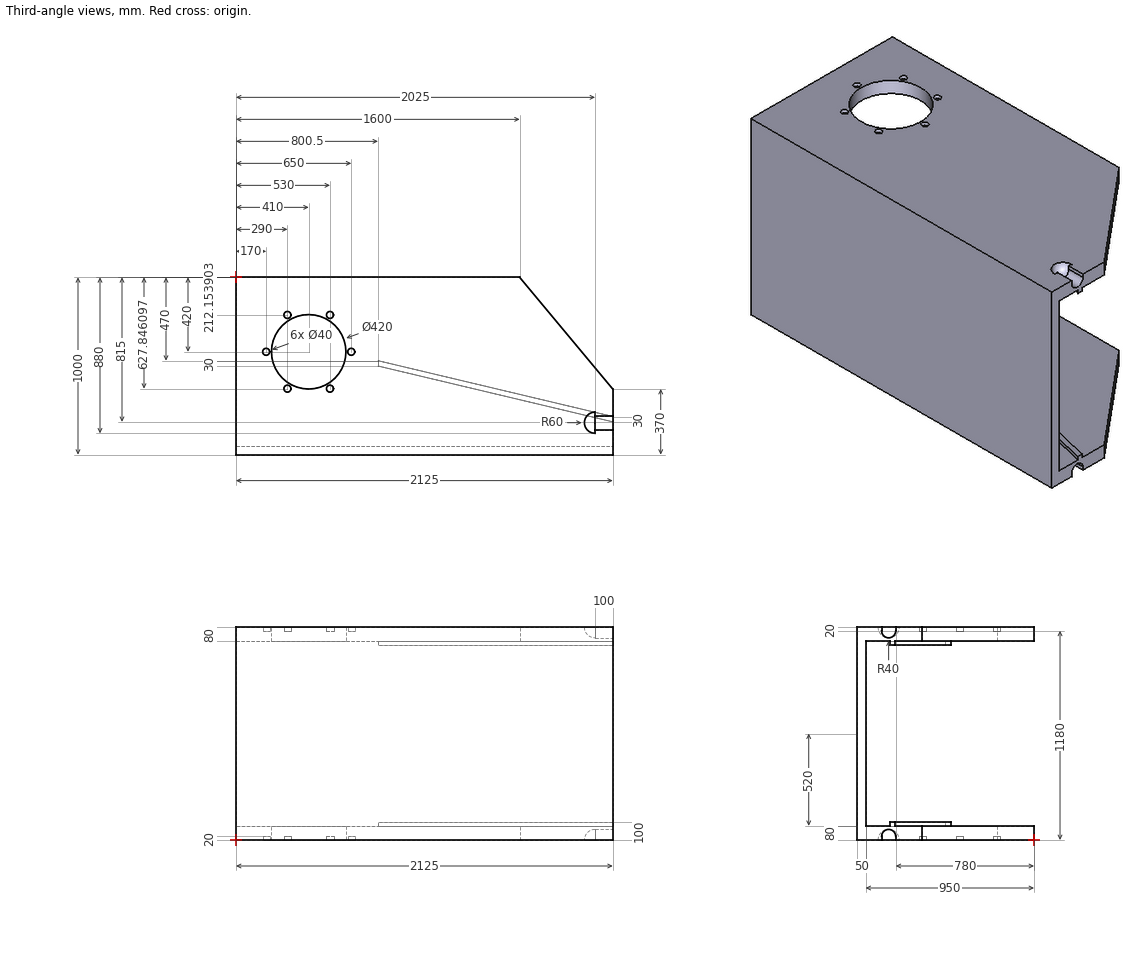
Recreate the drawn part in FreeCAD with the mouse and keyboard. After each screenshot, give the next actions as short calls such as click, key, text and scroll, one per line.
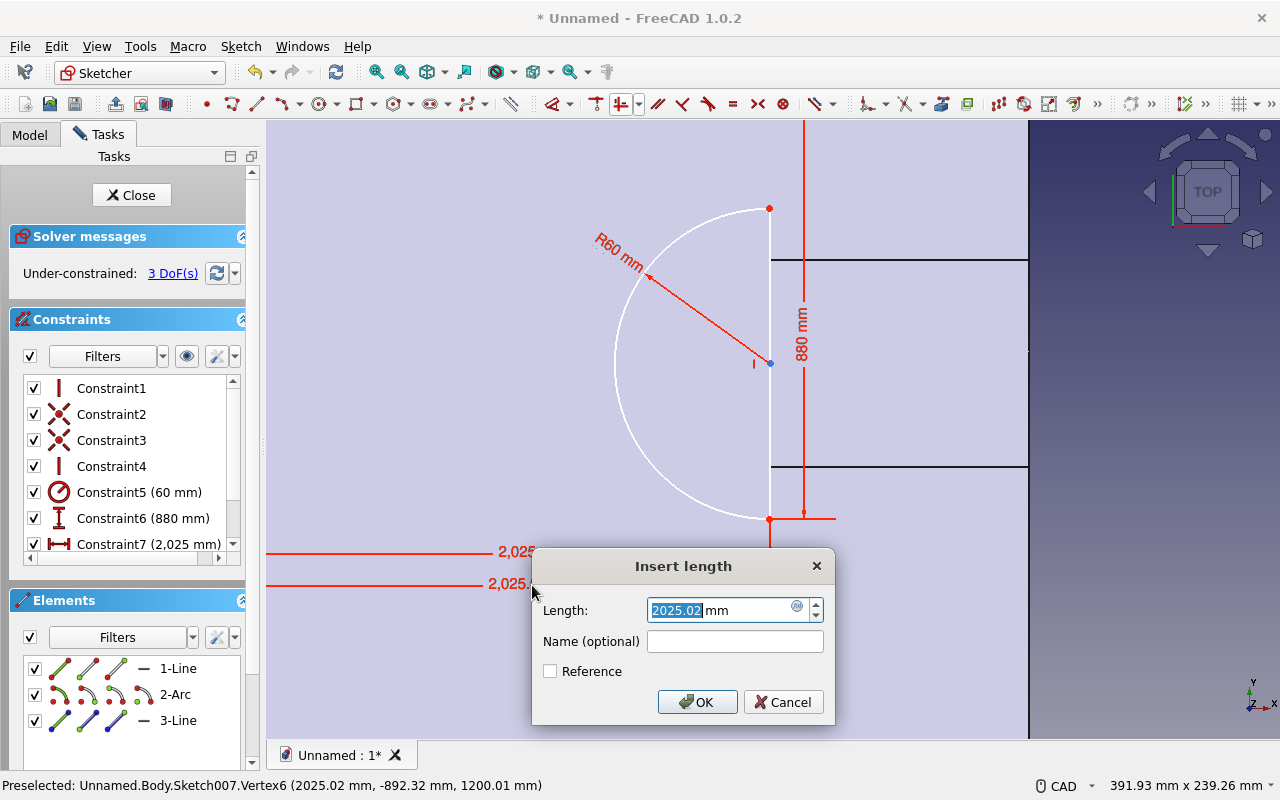
text(2025)
key(Return)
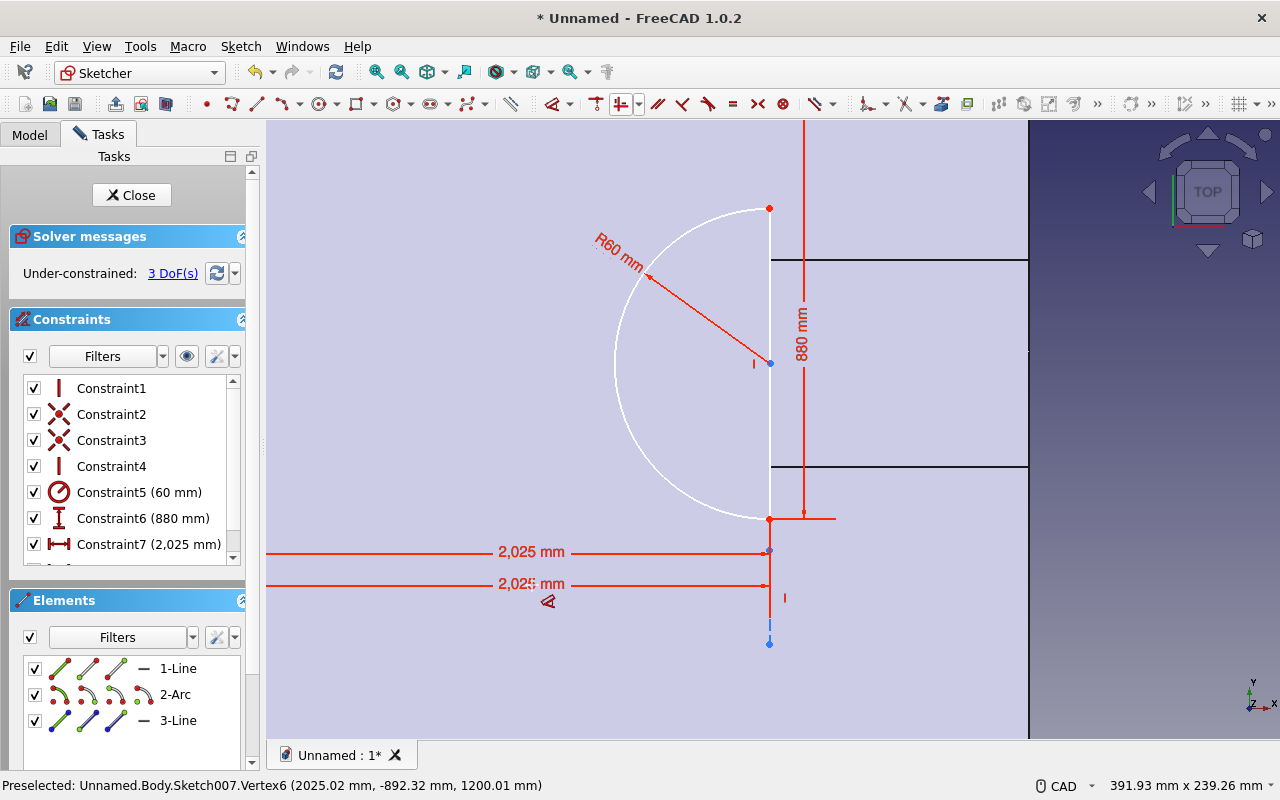
click(770, 364)
click(532, 398)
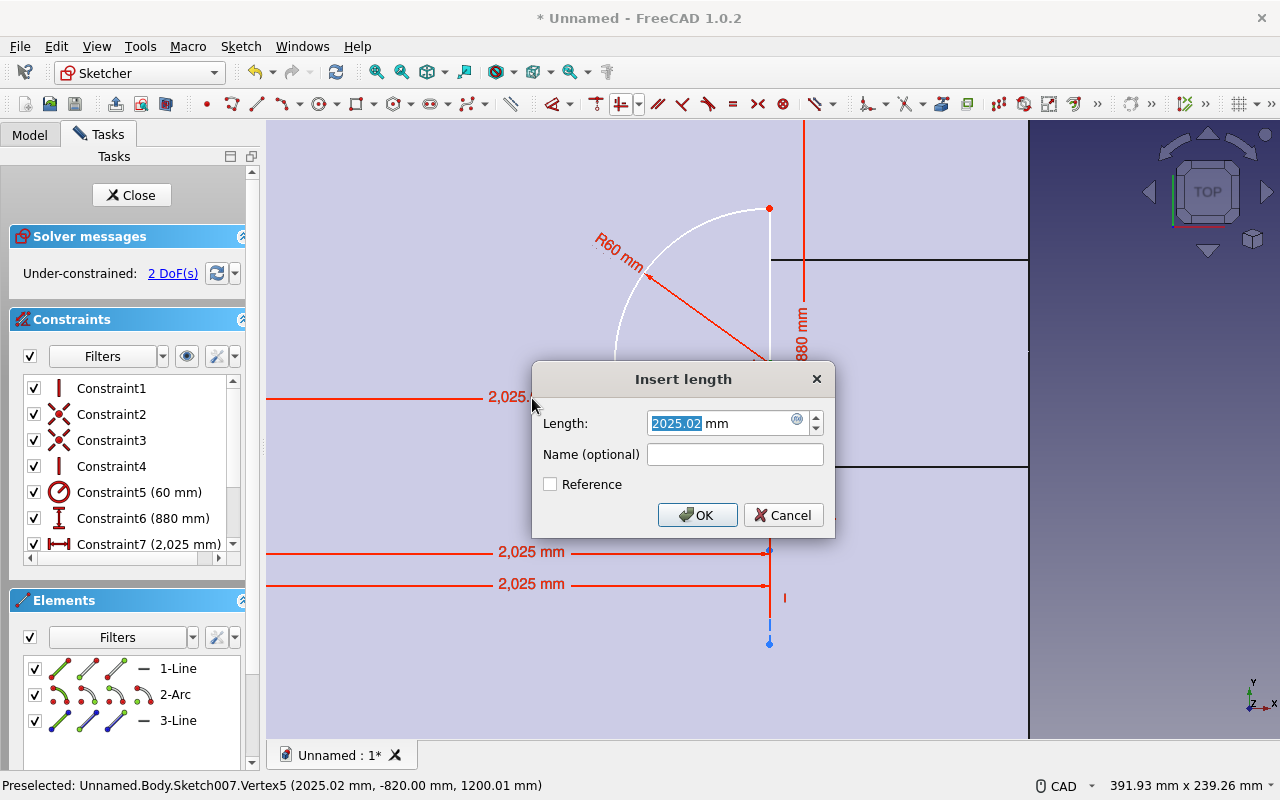
text(2025)
key(Return)
key(Escape)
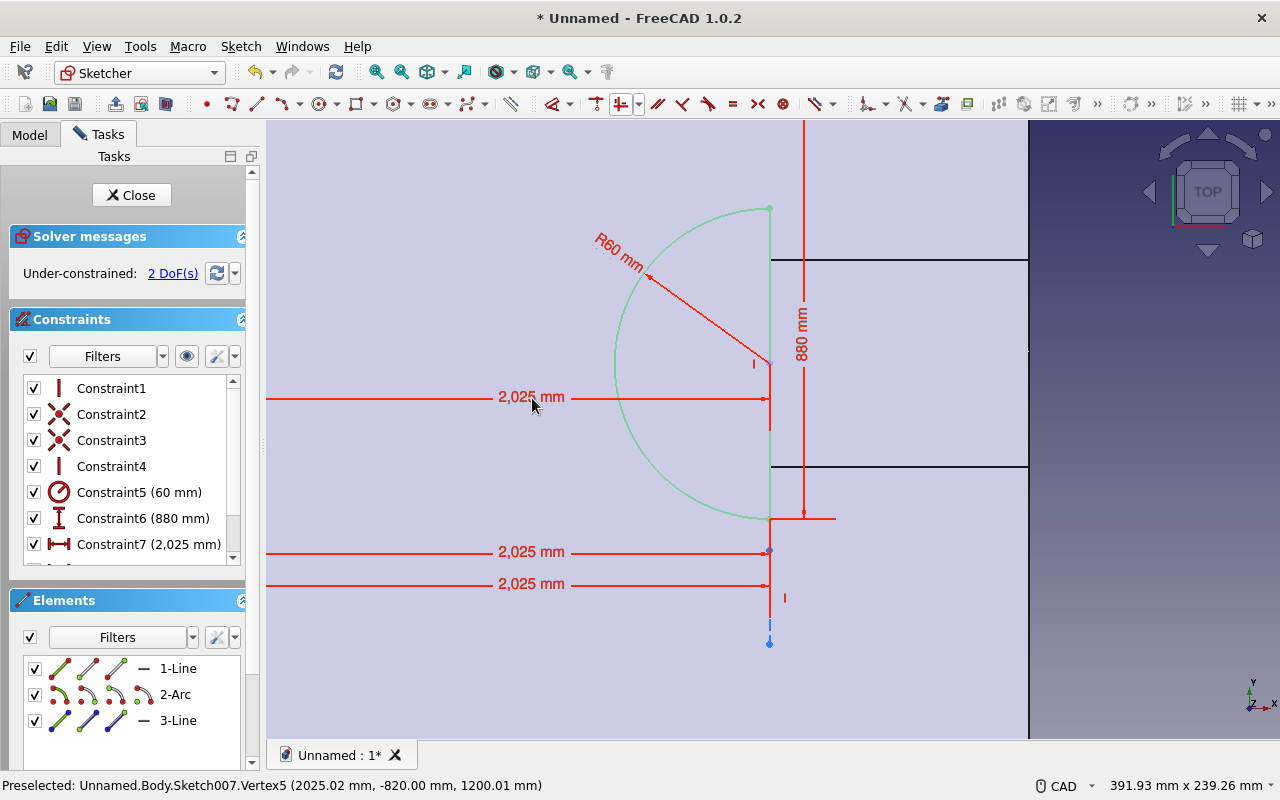
click(132, 195)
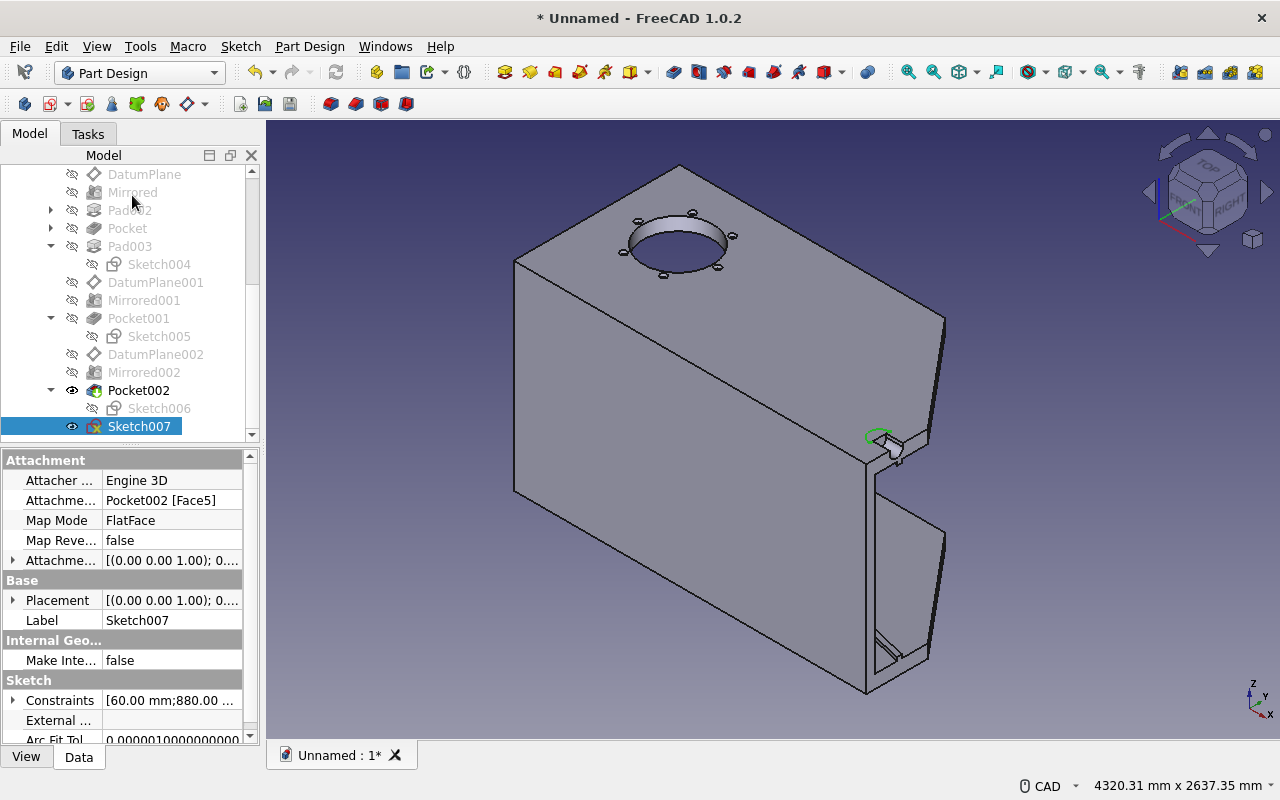
click(724, 72)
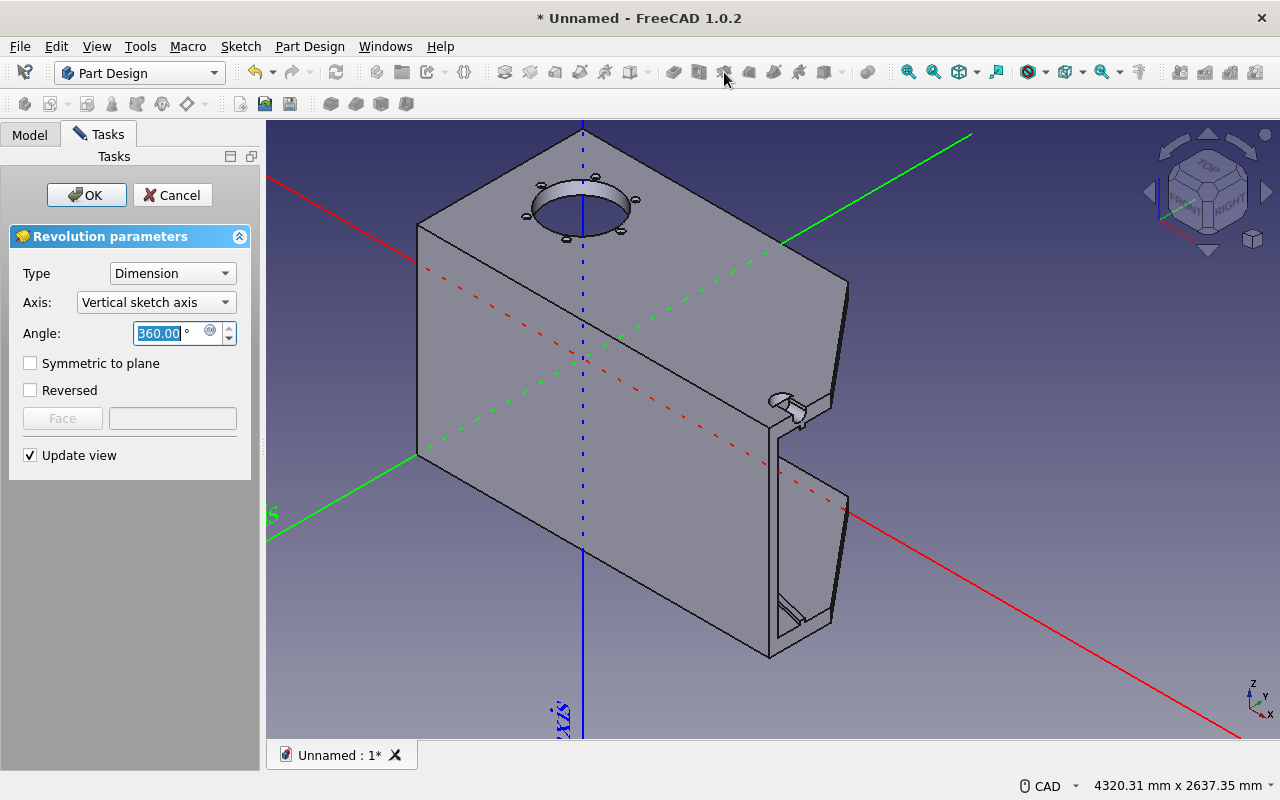
click(157, 302)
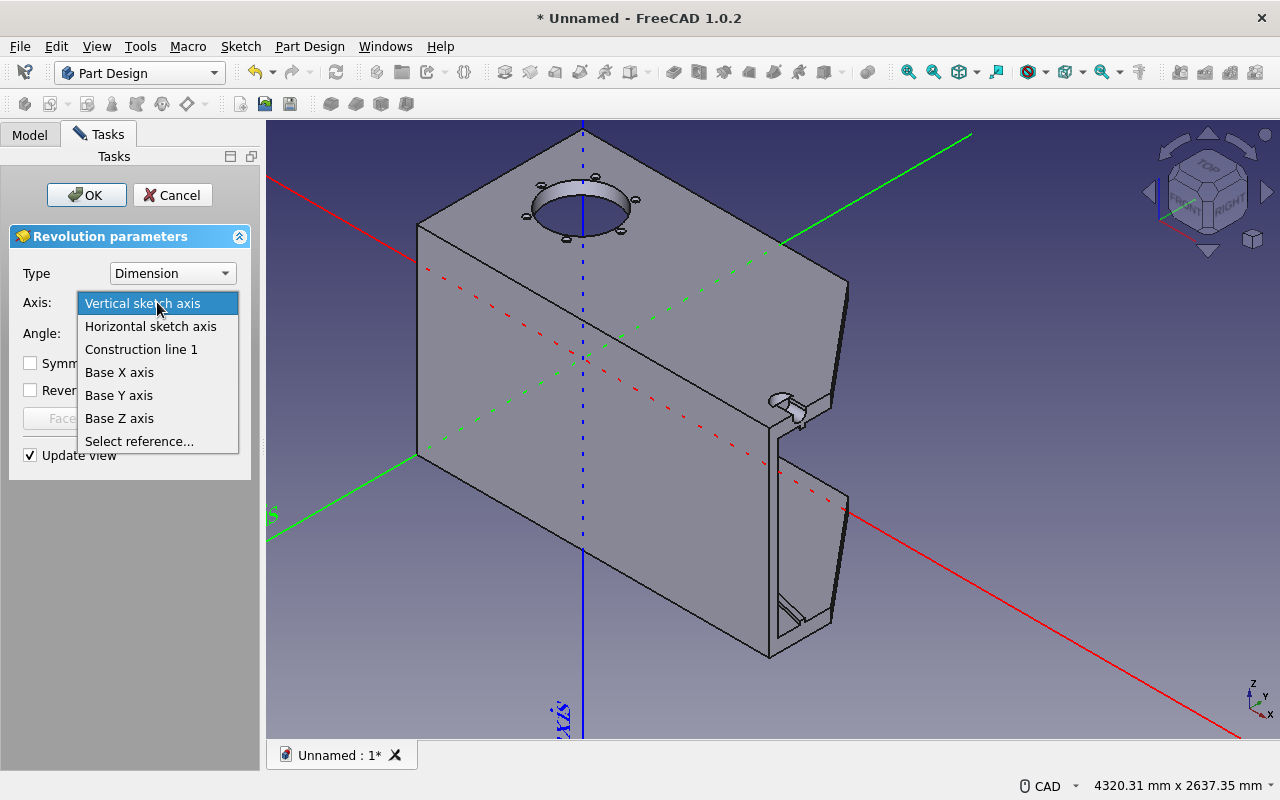
click(156, 350)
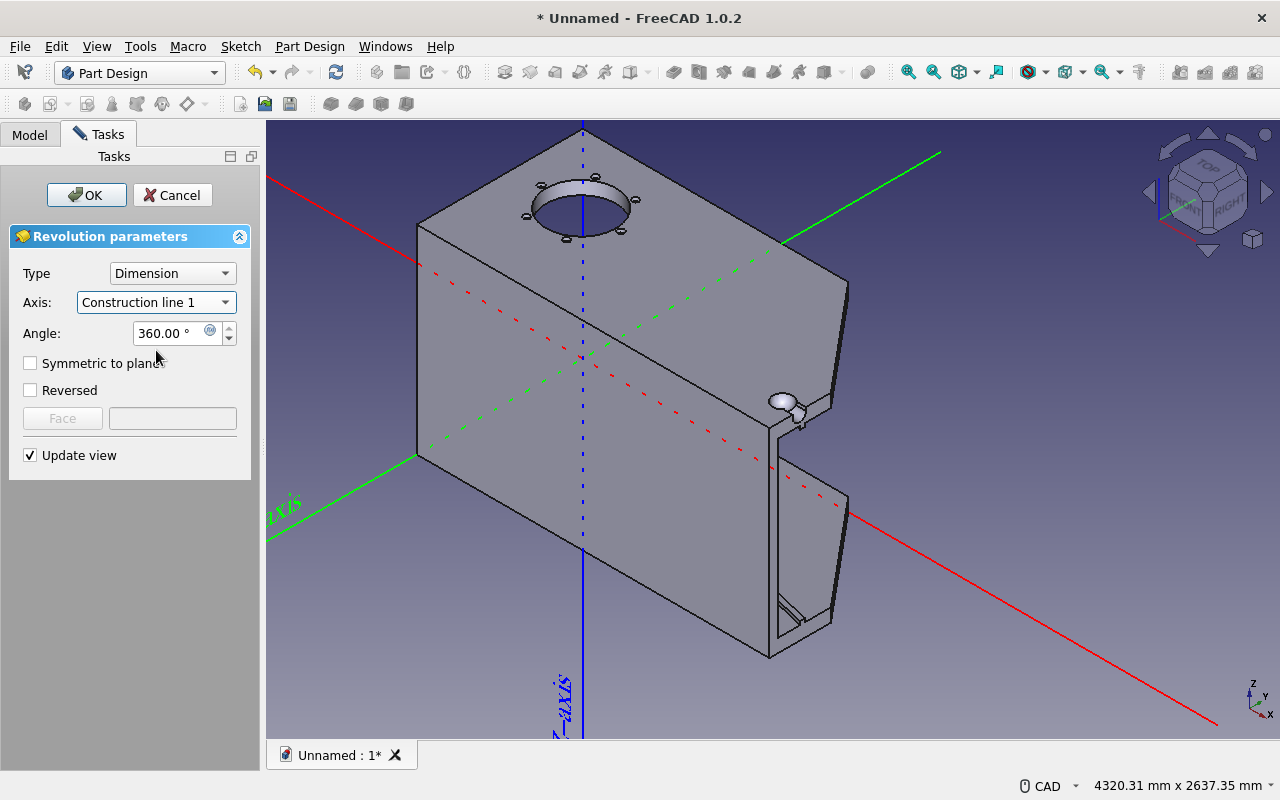
triple_click(178, 334)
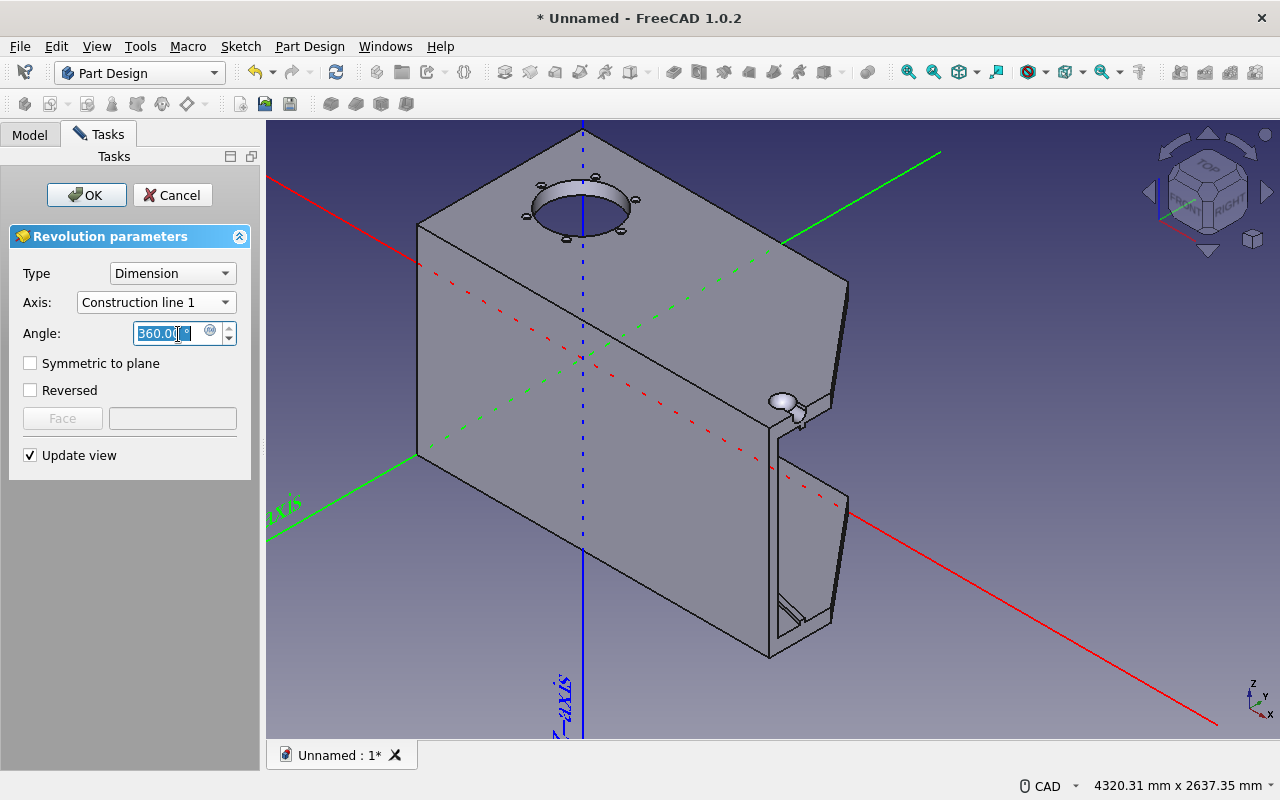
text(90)
key(Tab)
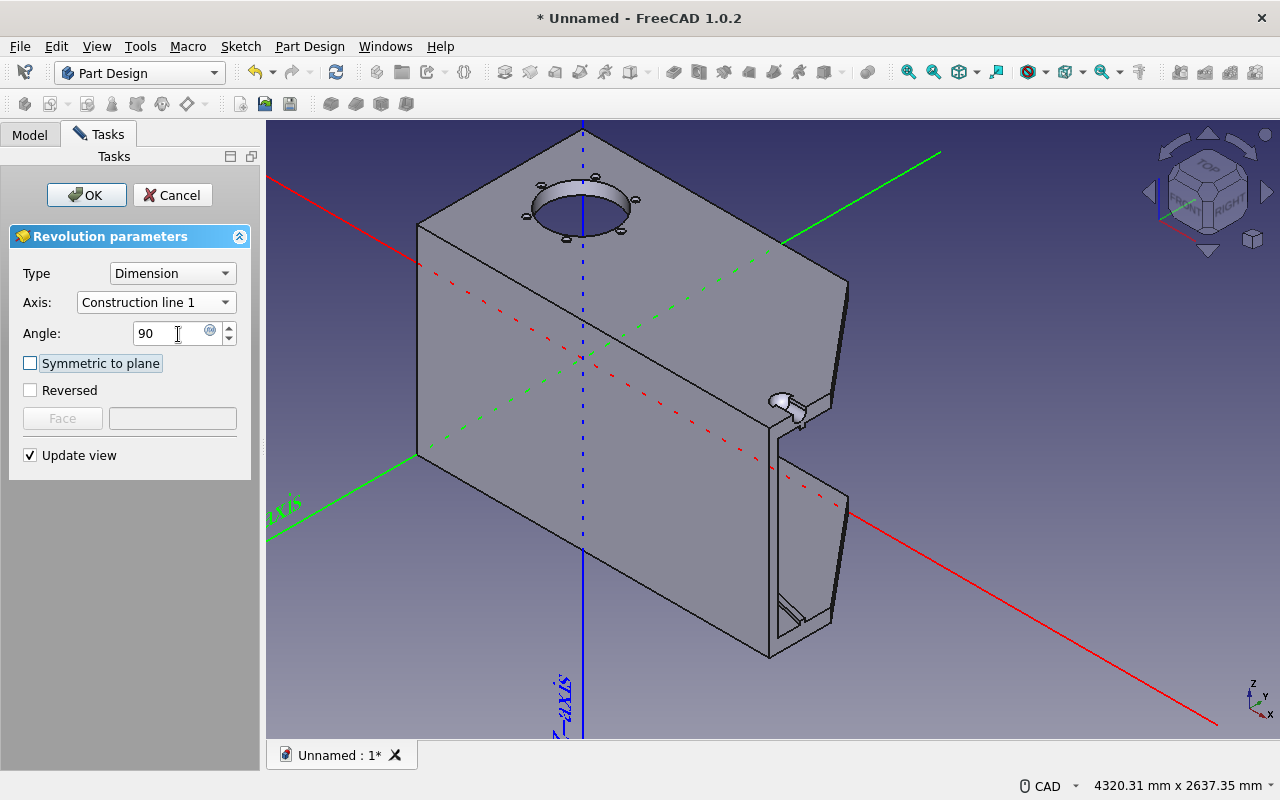
click(87, 195)